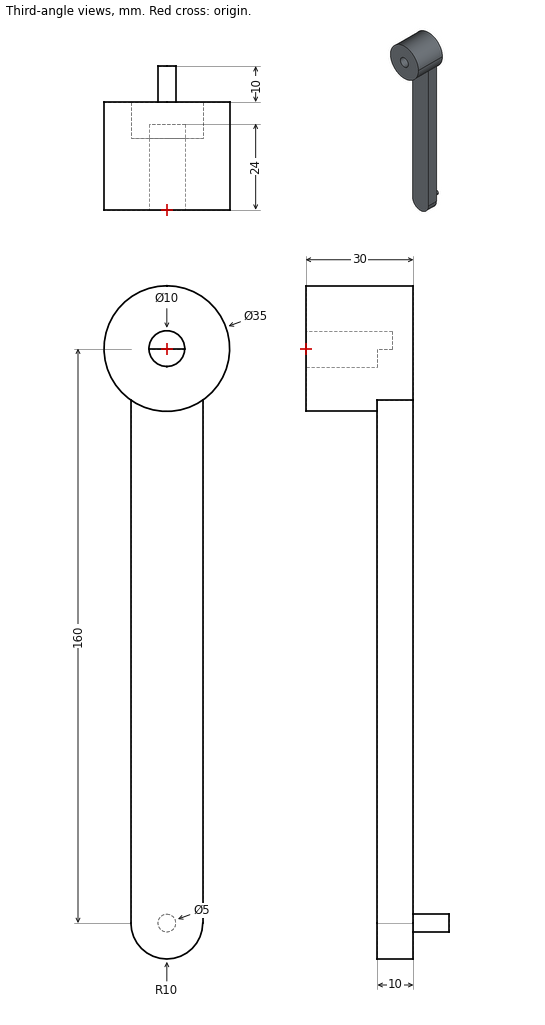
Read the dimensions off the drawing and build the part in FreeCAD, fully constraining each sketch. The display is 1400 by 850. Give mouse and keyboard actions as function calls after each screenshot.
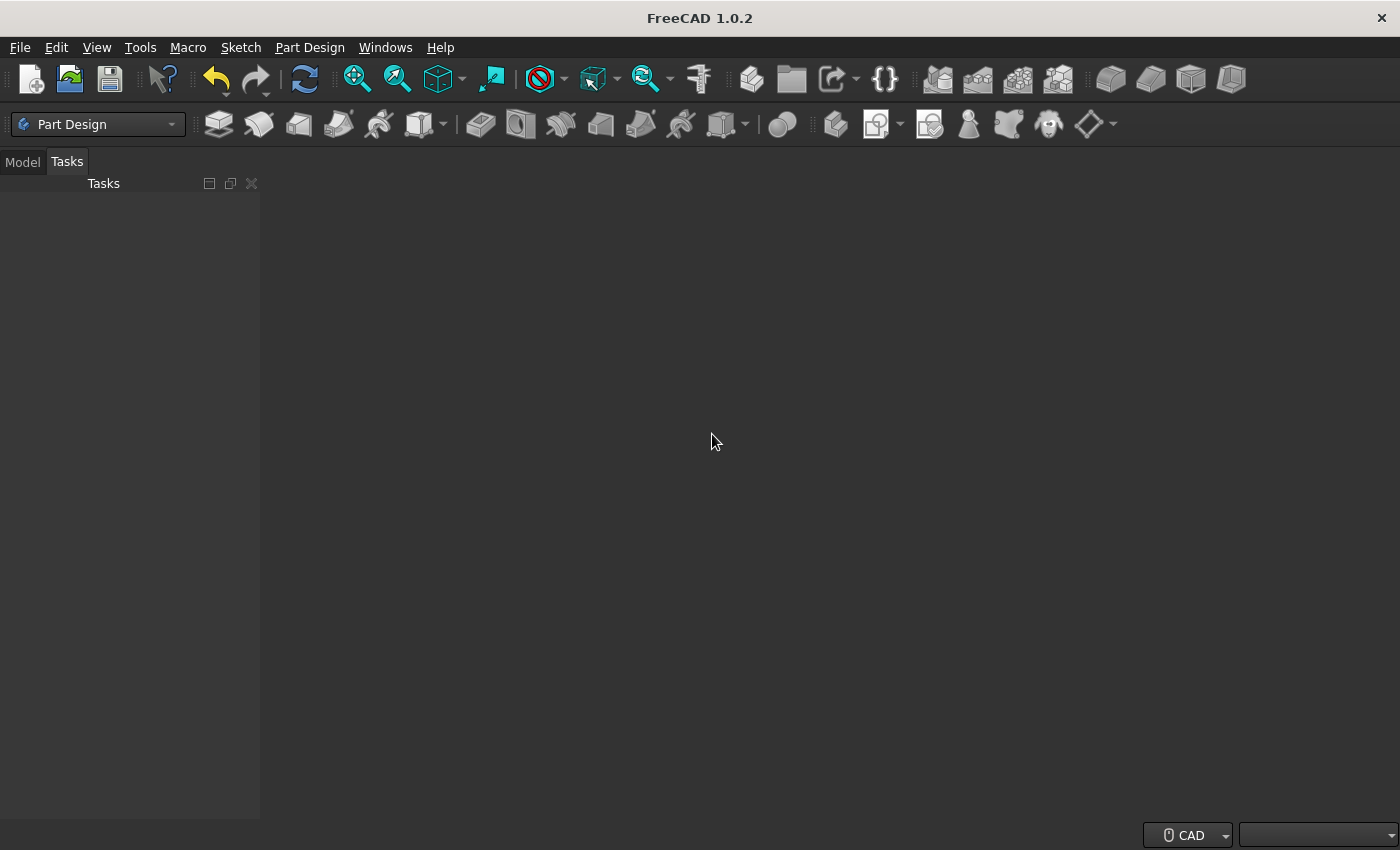
click(30, 80)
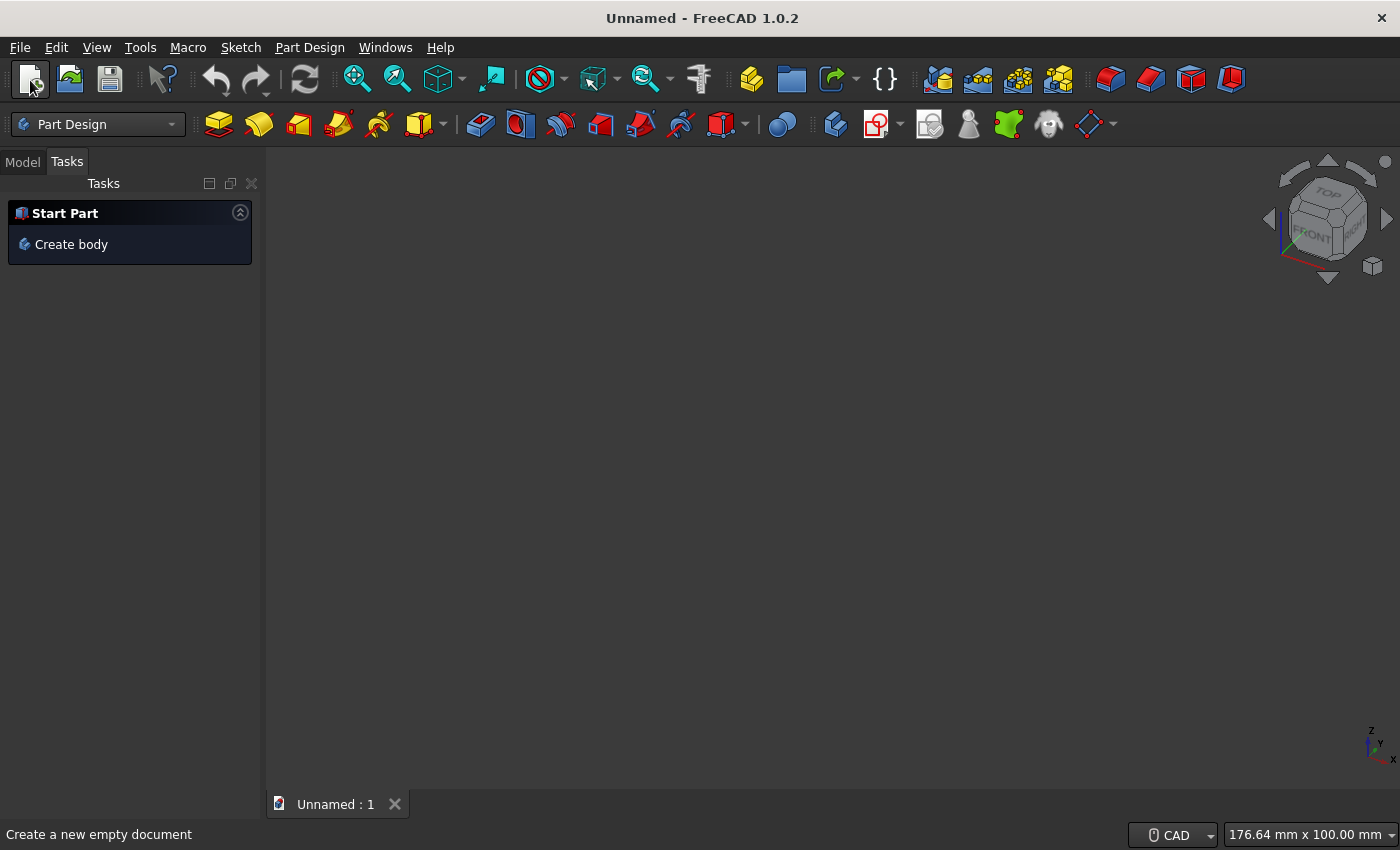
click(876, 124)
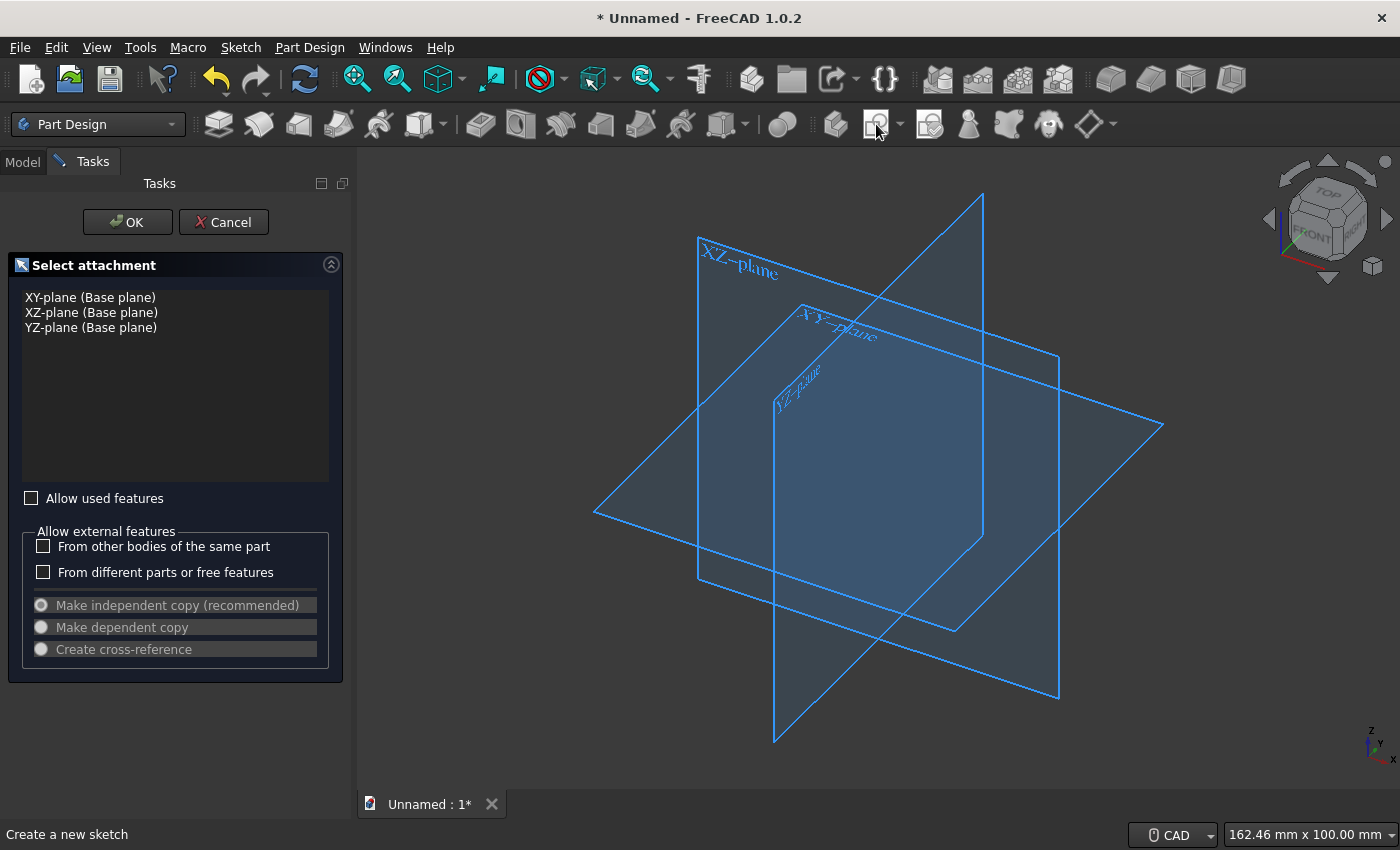
click(82, 312)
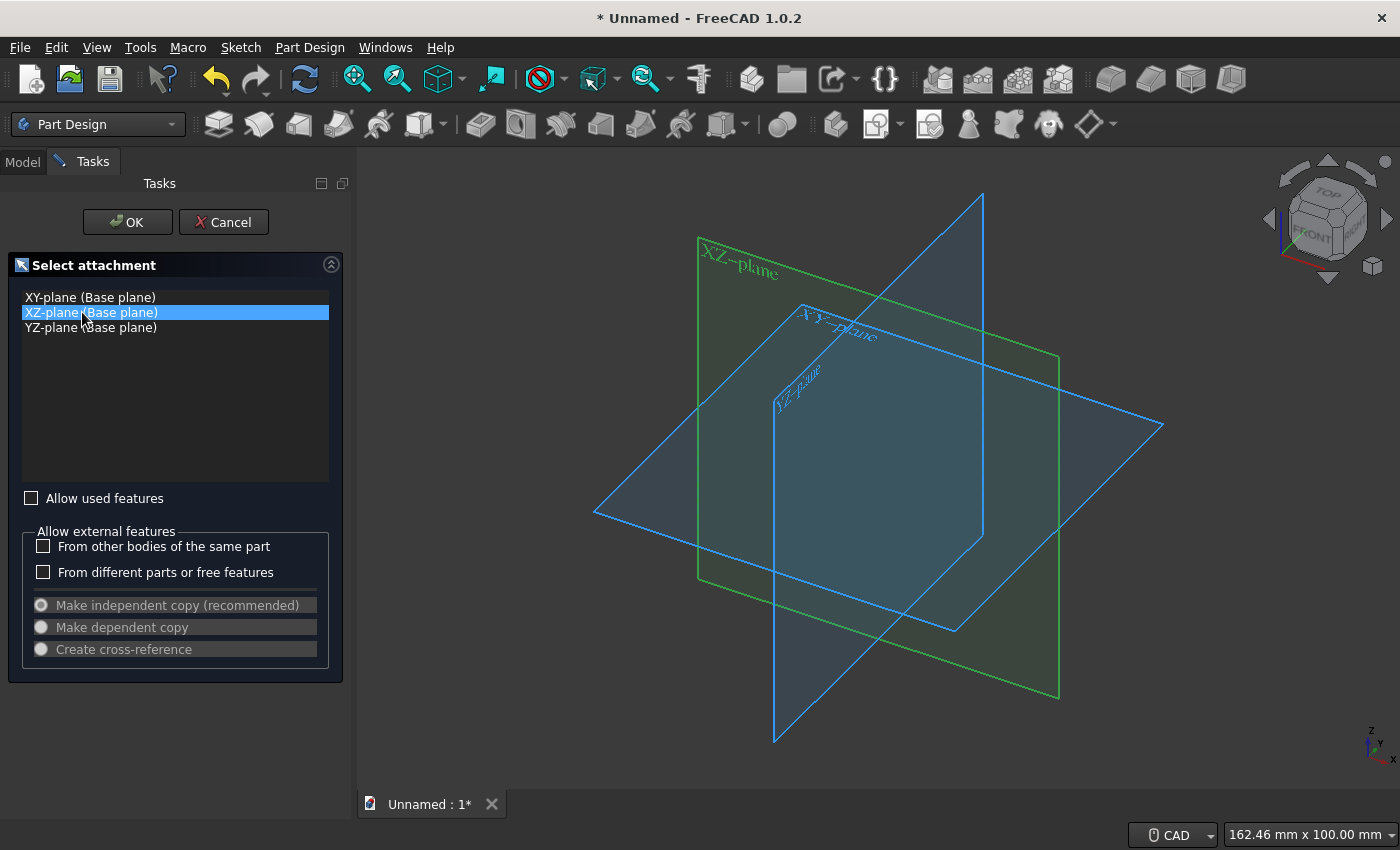
click(128, 222)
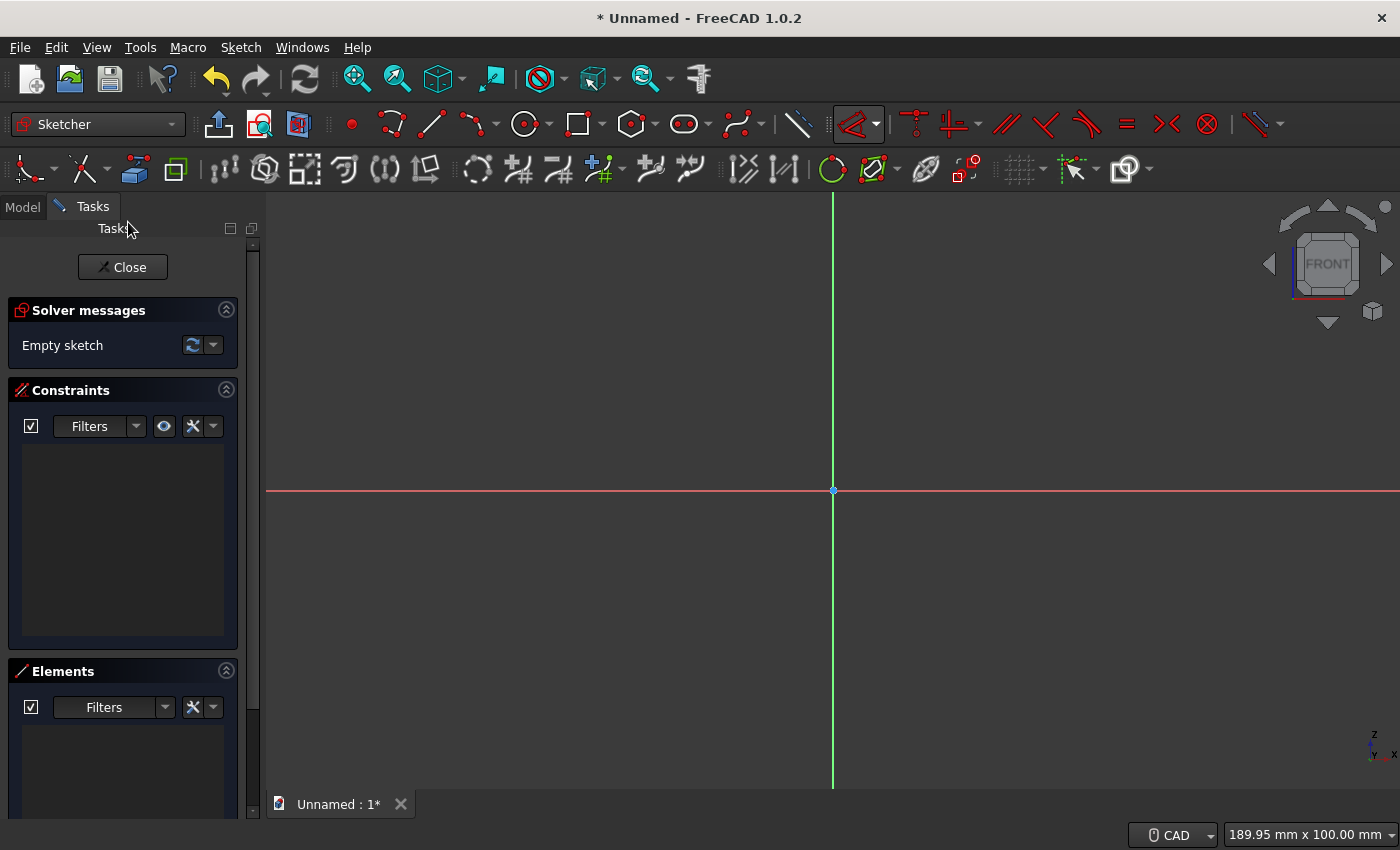
scroll(916, 490, up, 3)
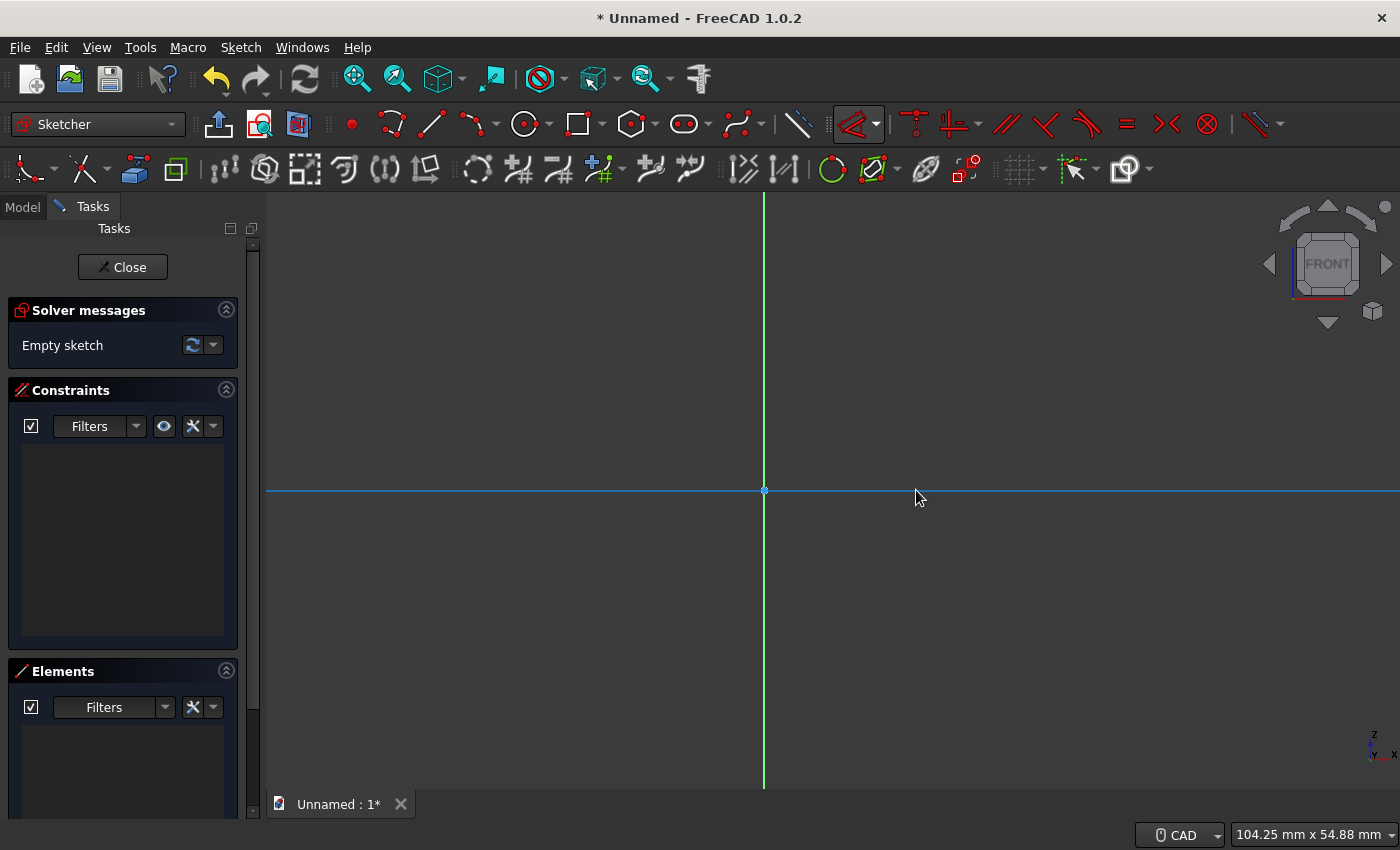
key(g)
key(c)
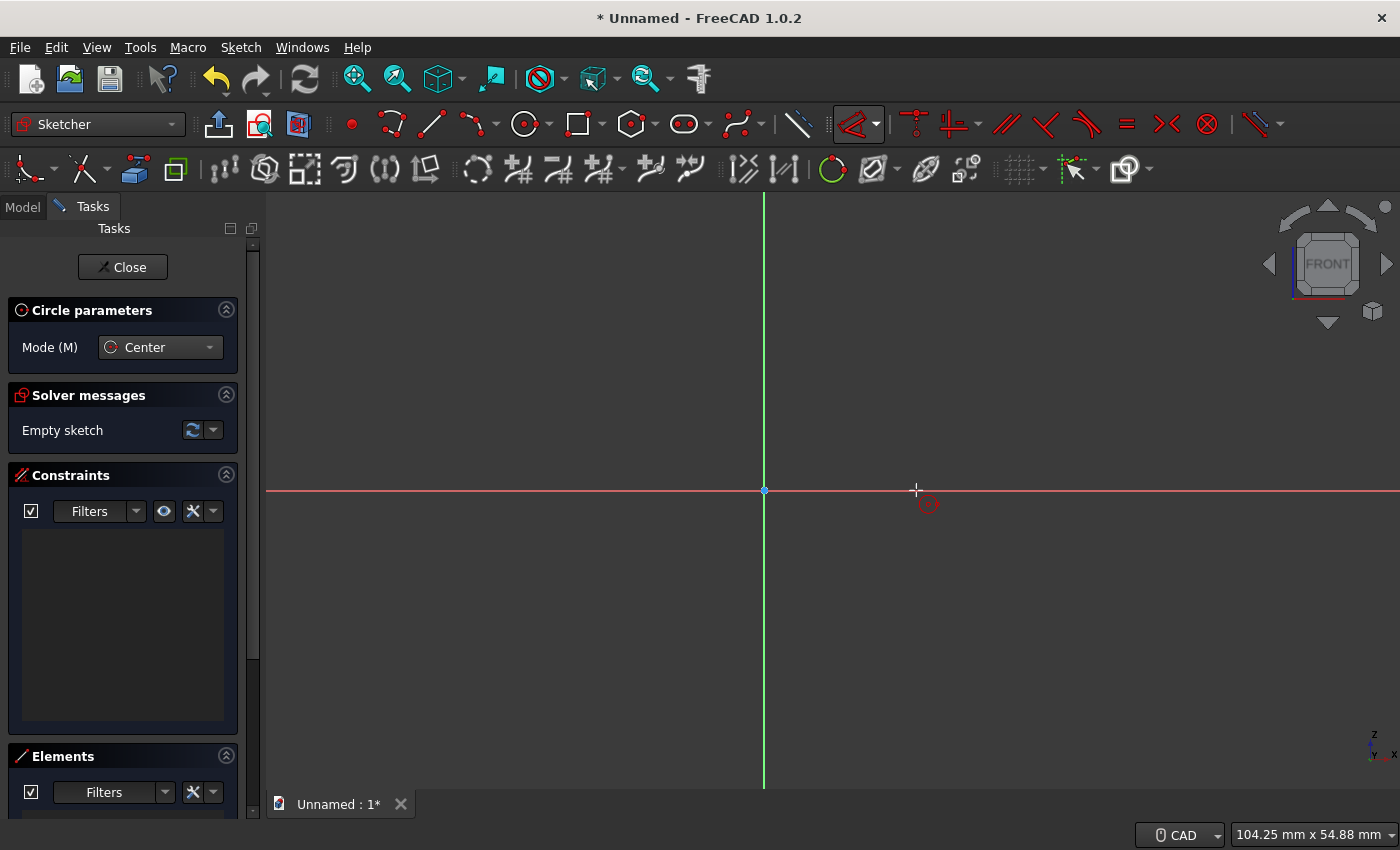
click(764, 490)
move(899, 356)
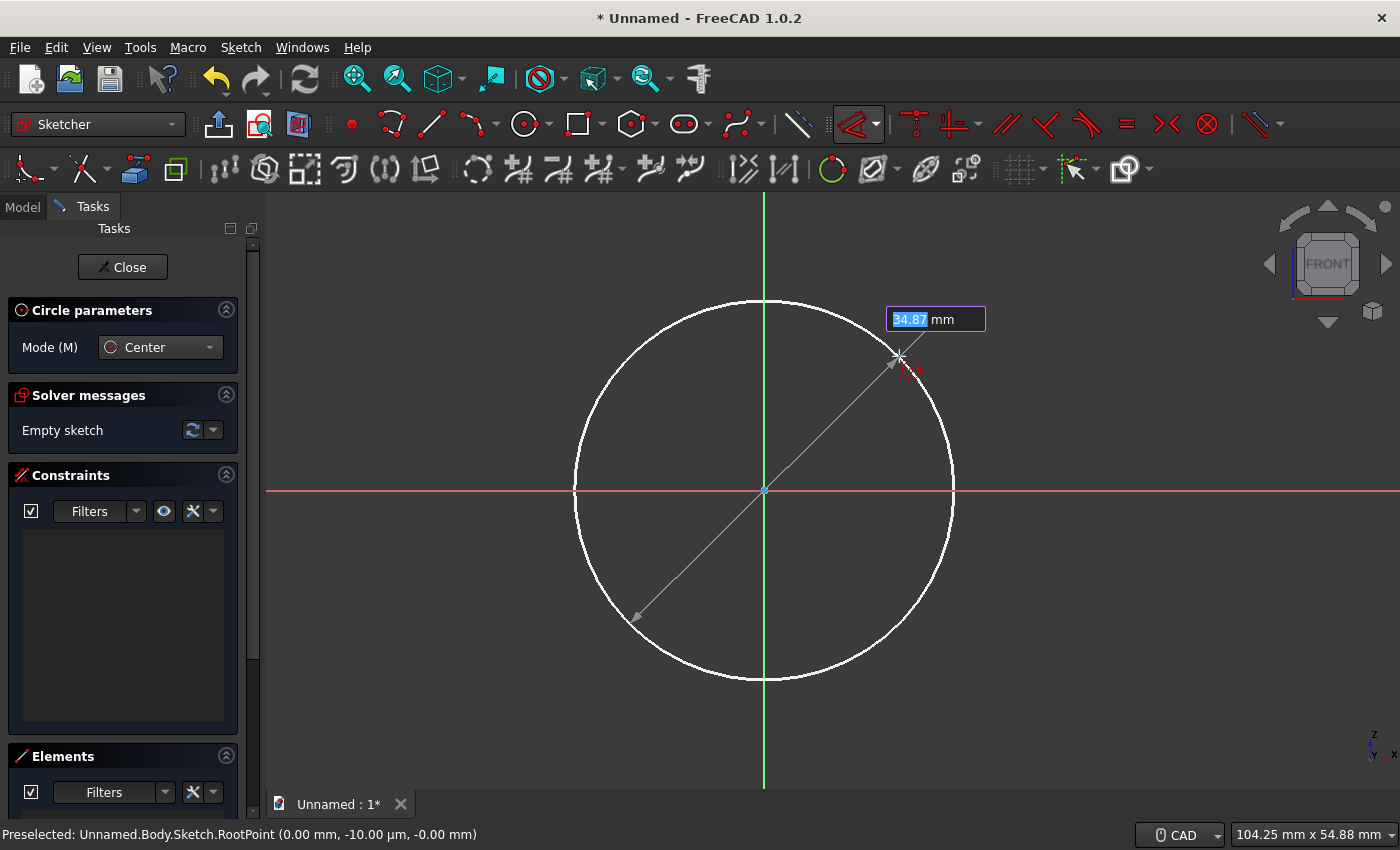
text(35)
key(Return)
key(Escape)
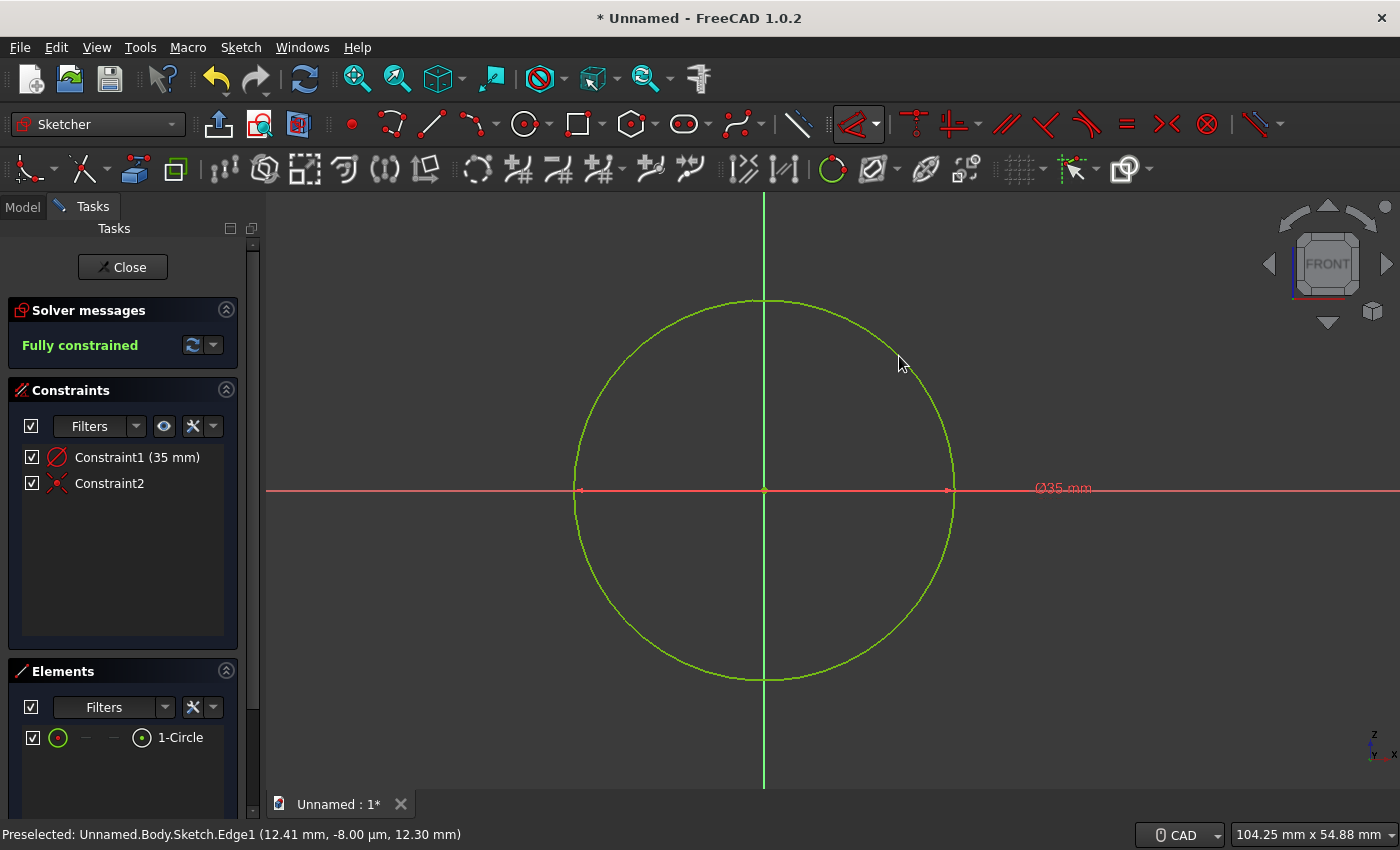
click(123, 267)